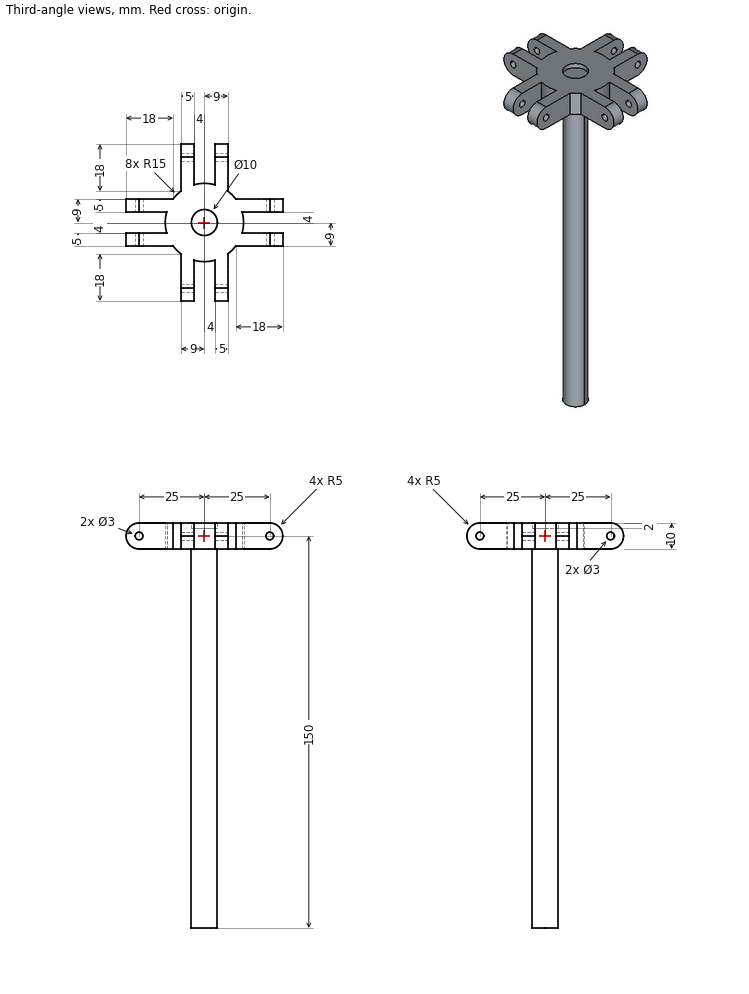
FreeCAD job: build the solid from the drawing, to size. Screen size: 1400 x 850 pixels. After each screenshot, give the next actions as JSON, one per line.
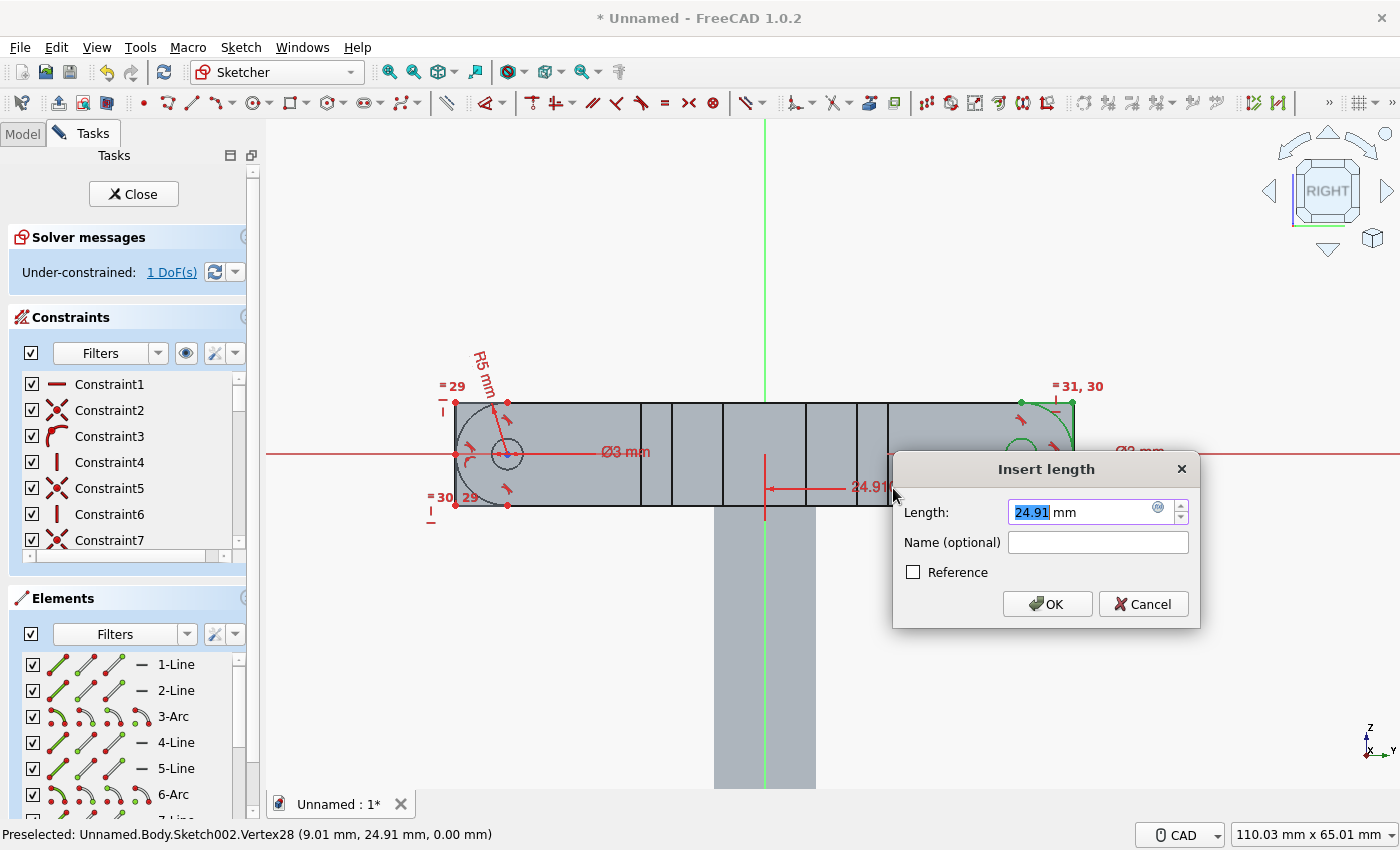
{"action": "type", "text": "25"}
{"action": "key", "text": "Return"}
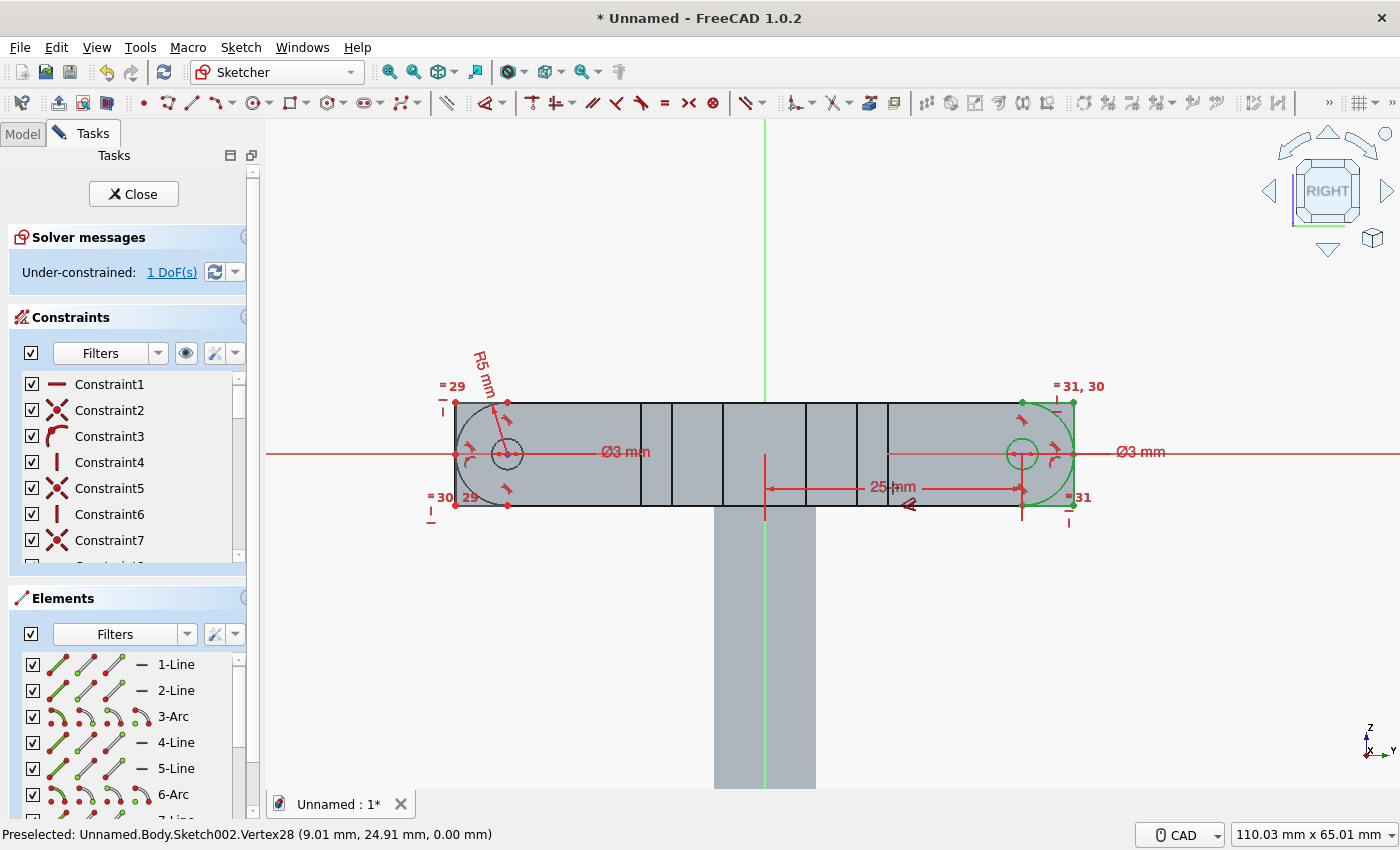
{"action": "left_click", "coordinate": [507, 454]}
{"action": "left_click", "coordinate": [636, 488]}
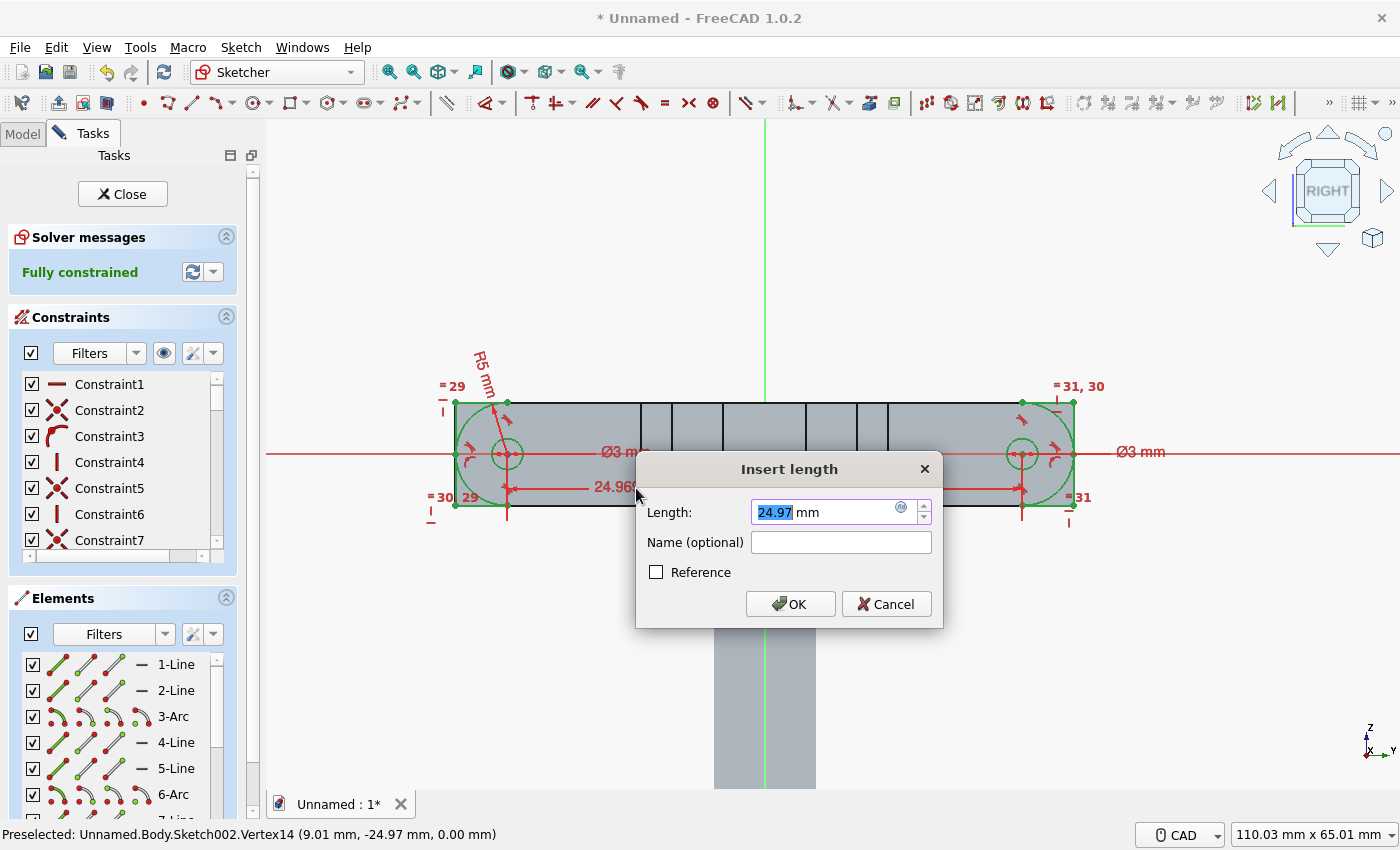
{"action": "type", "text": "25"}
{"action": "key", "text": "Return"}
{"action": "key", "text": "Escape"}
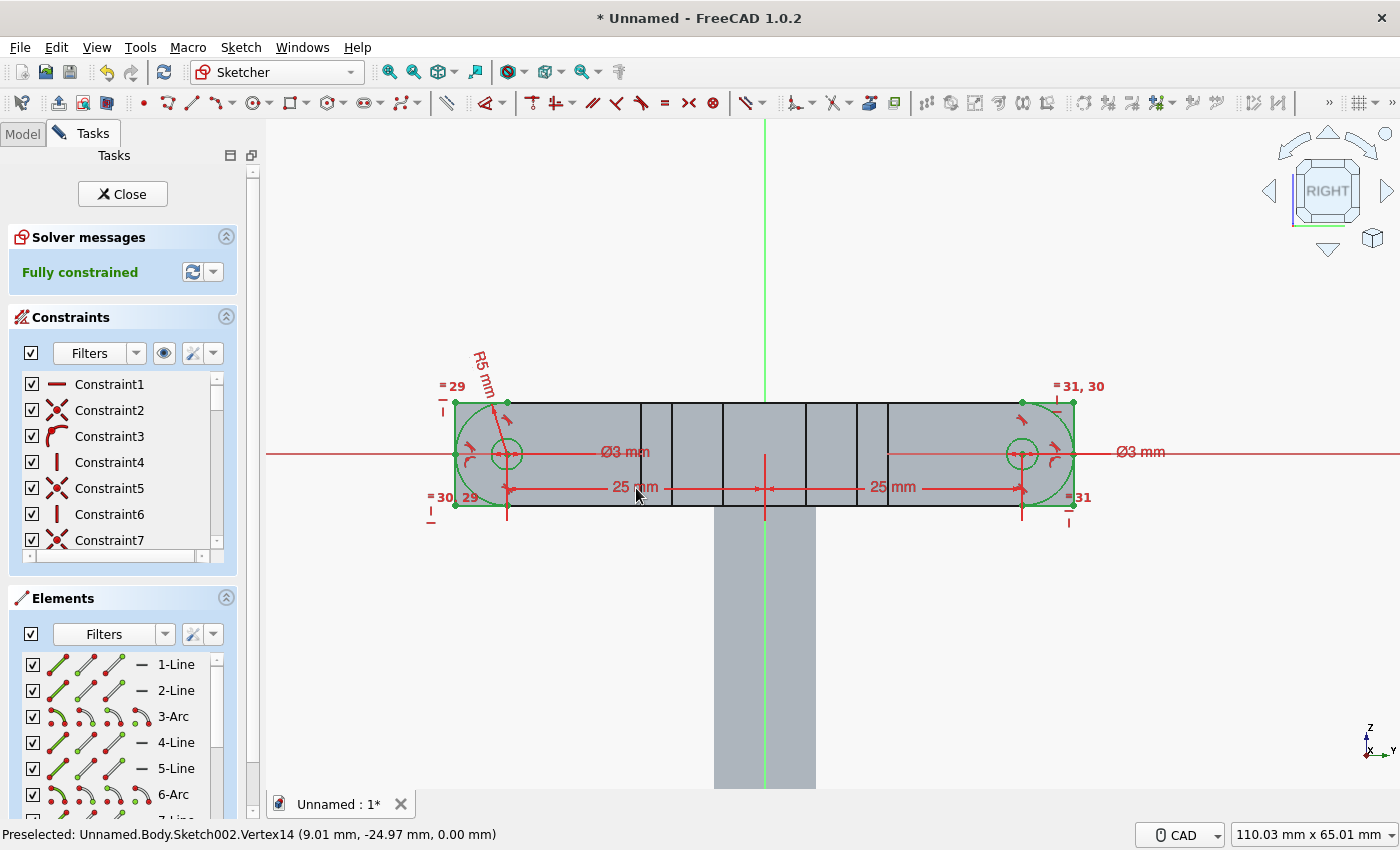
{"action": "left_click", "coordinate": [123, 194]}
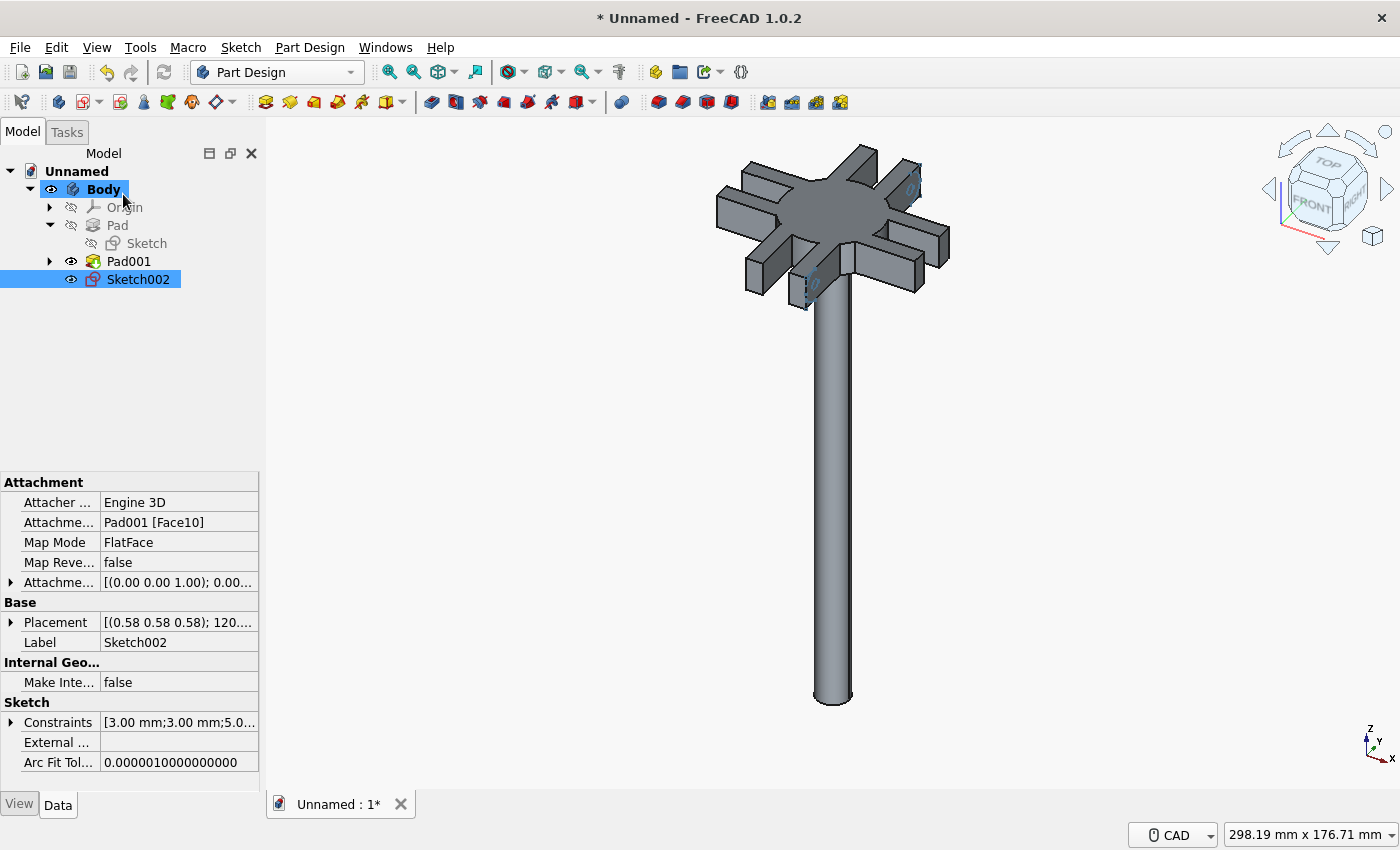
{"action": "left_click", "coordinate": [432, 102]}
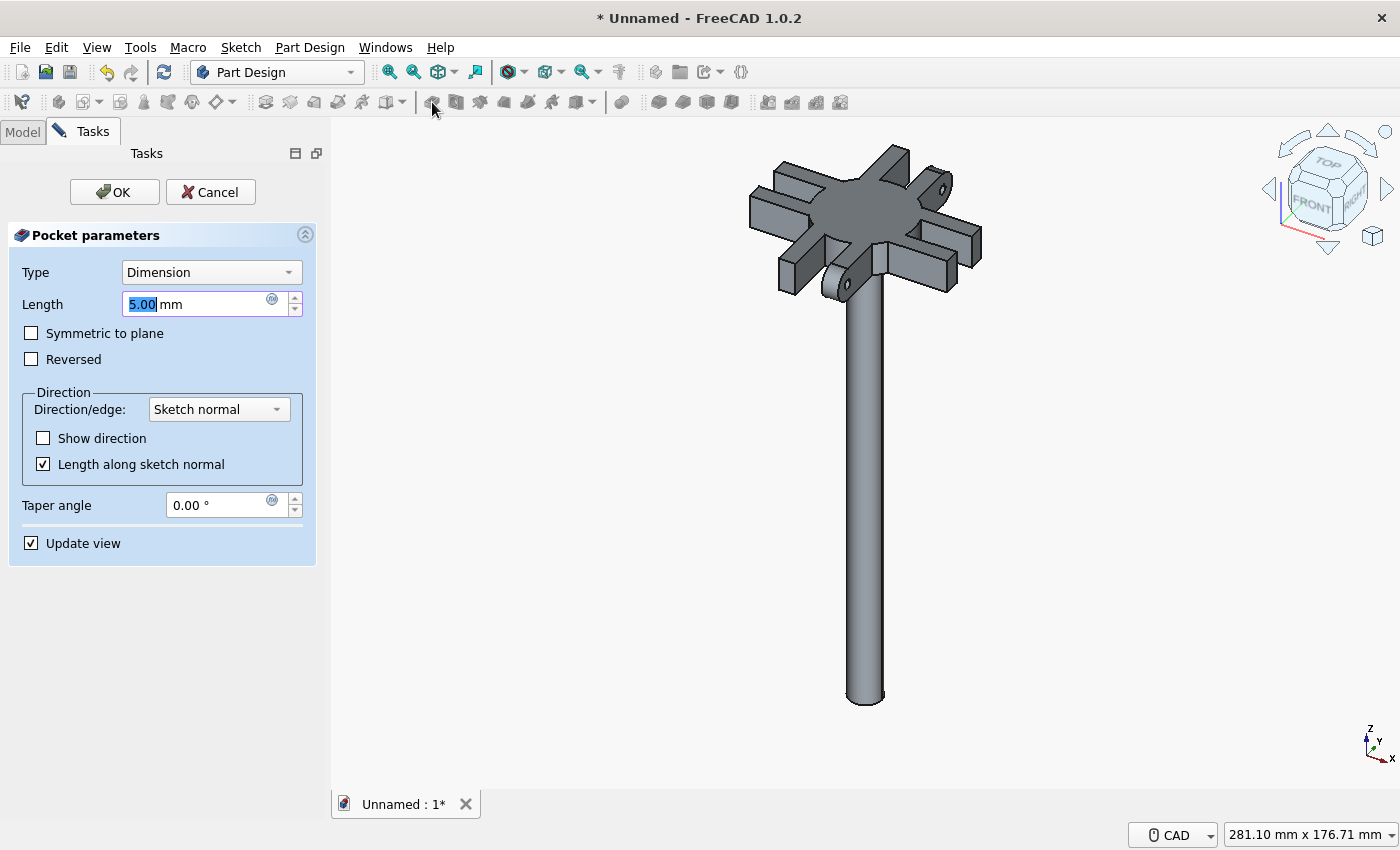
{"action": "left_click", "coordinate": [212, 272]}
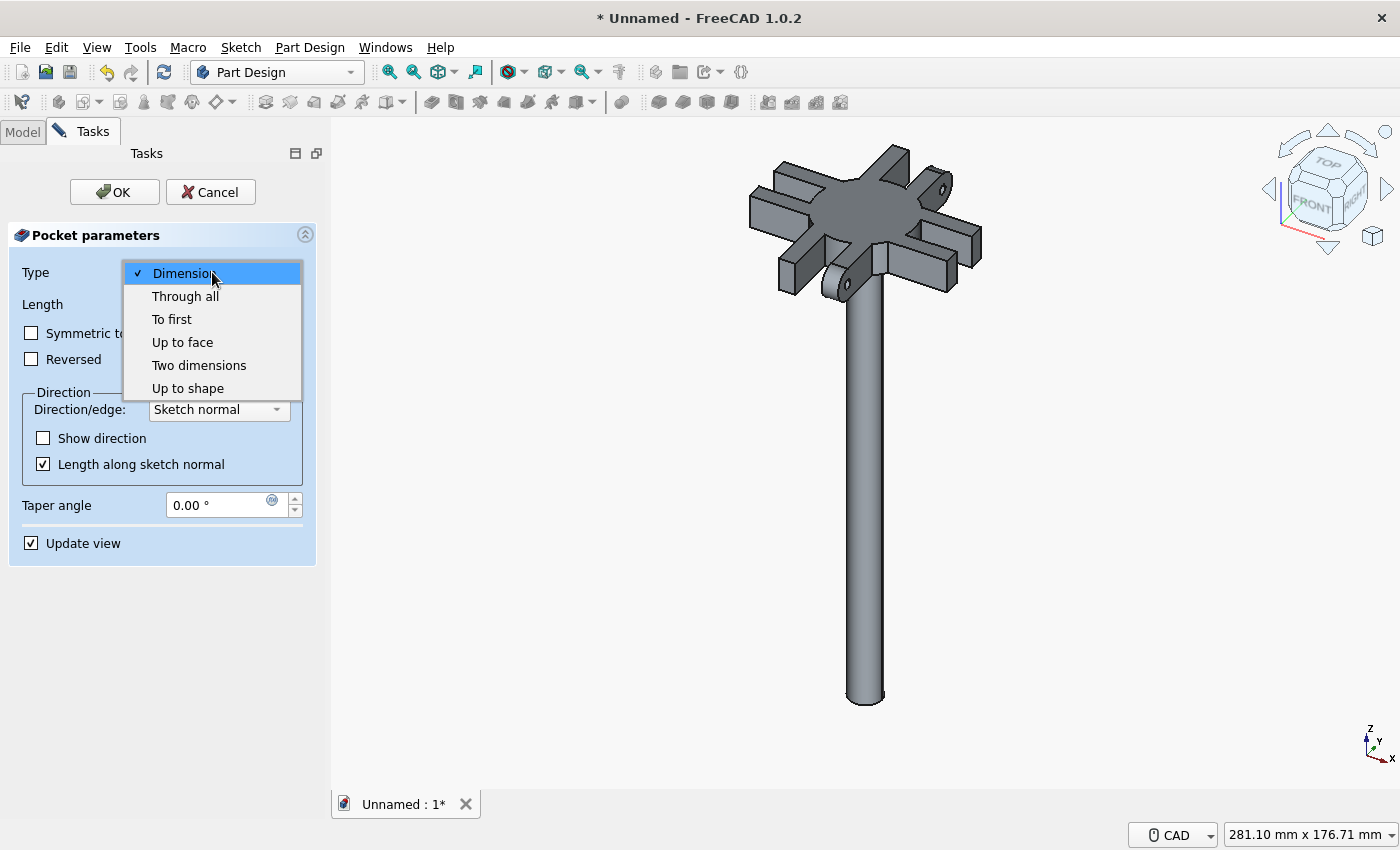
{"action": "left_click", "coordinate": [212, 296]}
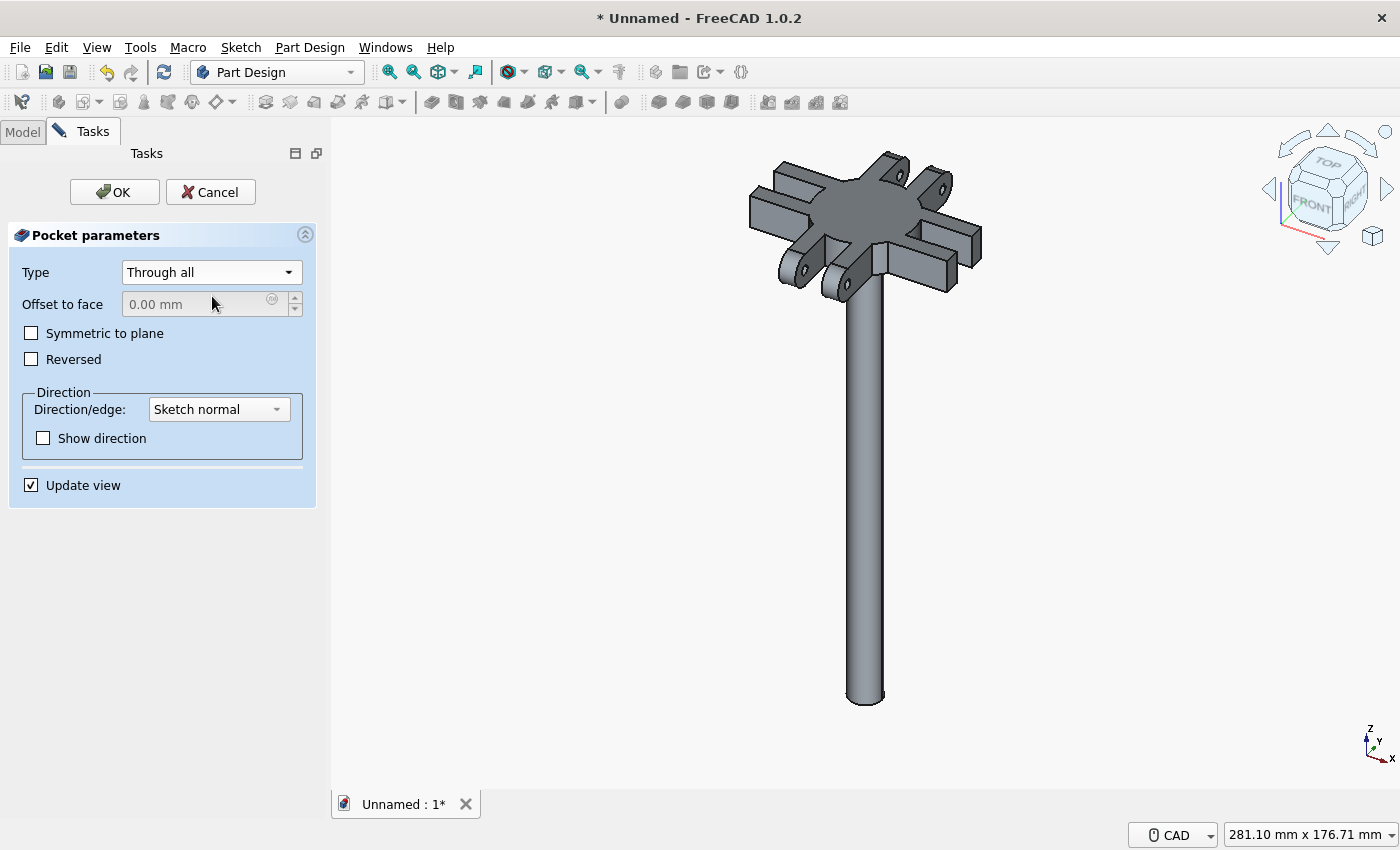
{"action": "left_click", "coordinate": [115, 192]}